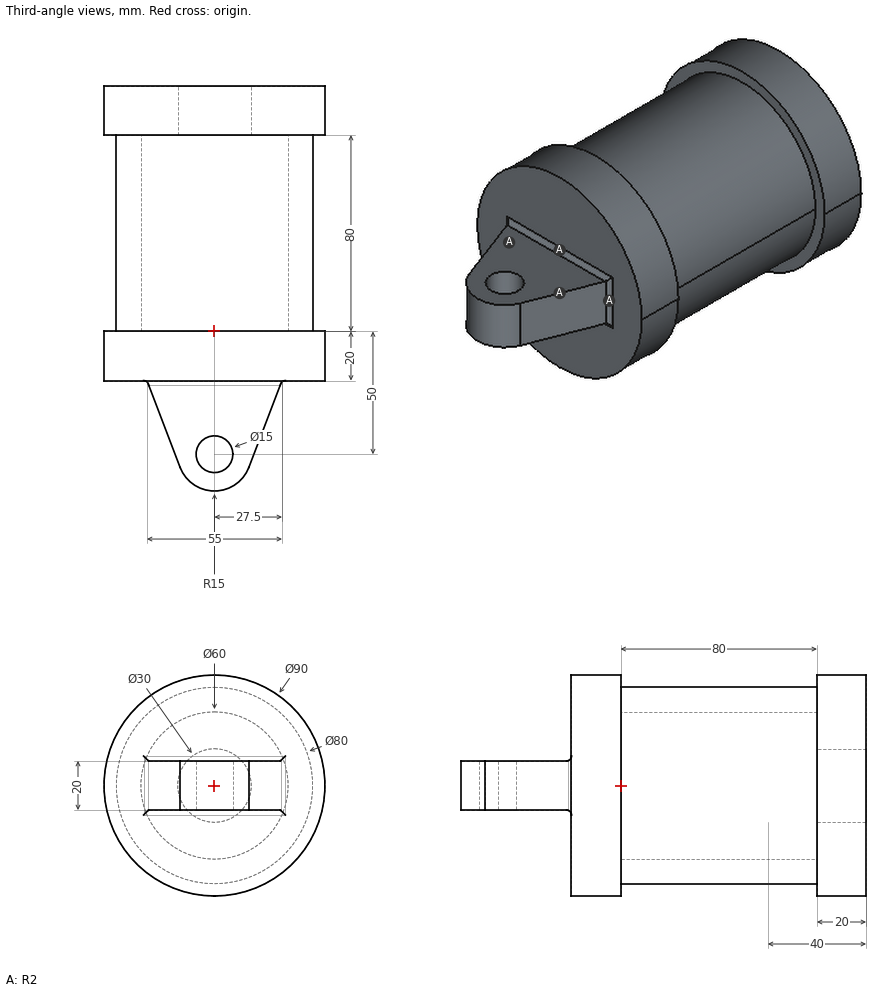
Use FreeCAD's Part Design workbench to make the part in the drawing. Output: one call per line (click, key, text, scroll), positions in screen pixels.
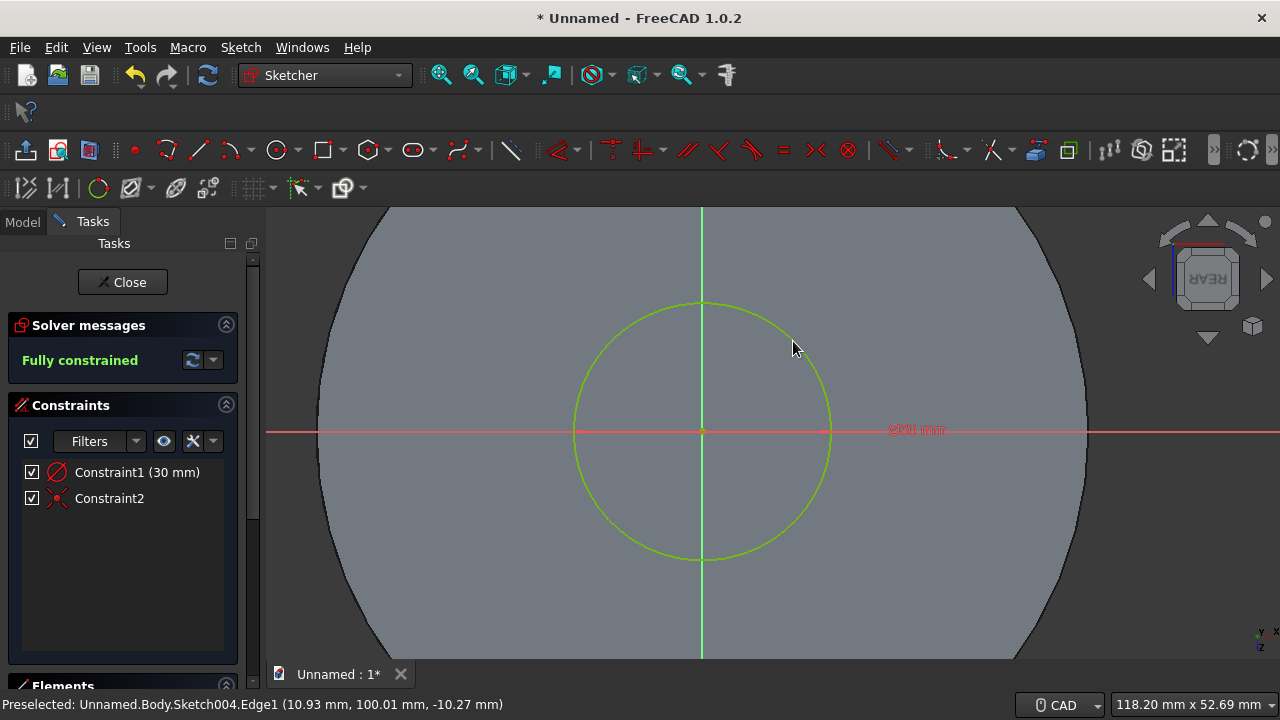
click(123, 282)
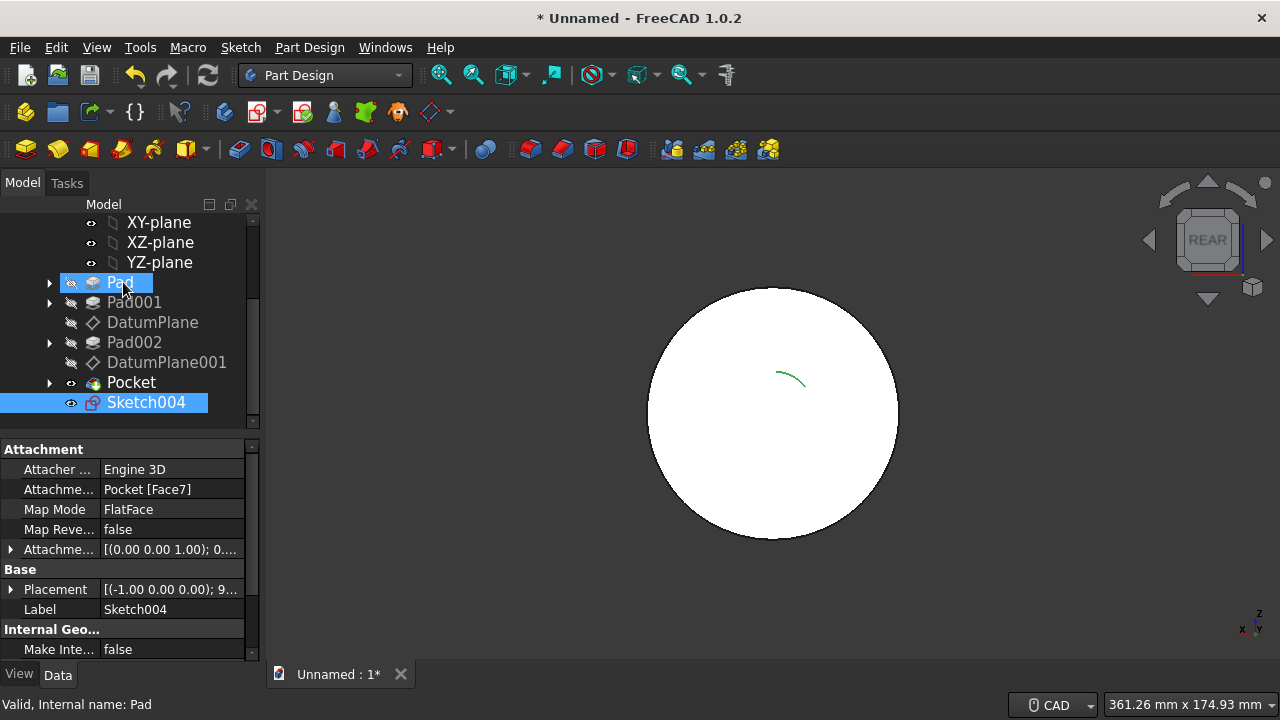
click(240, 150)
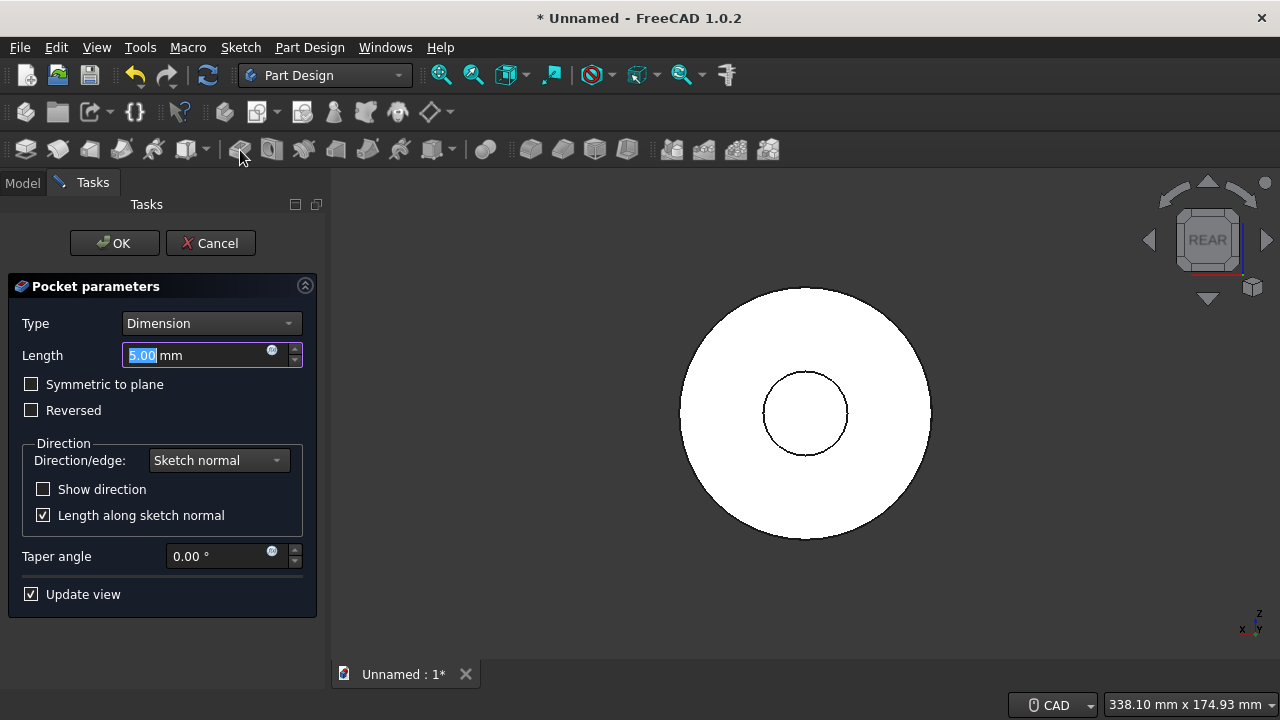
text(40)
key(Tab)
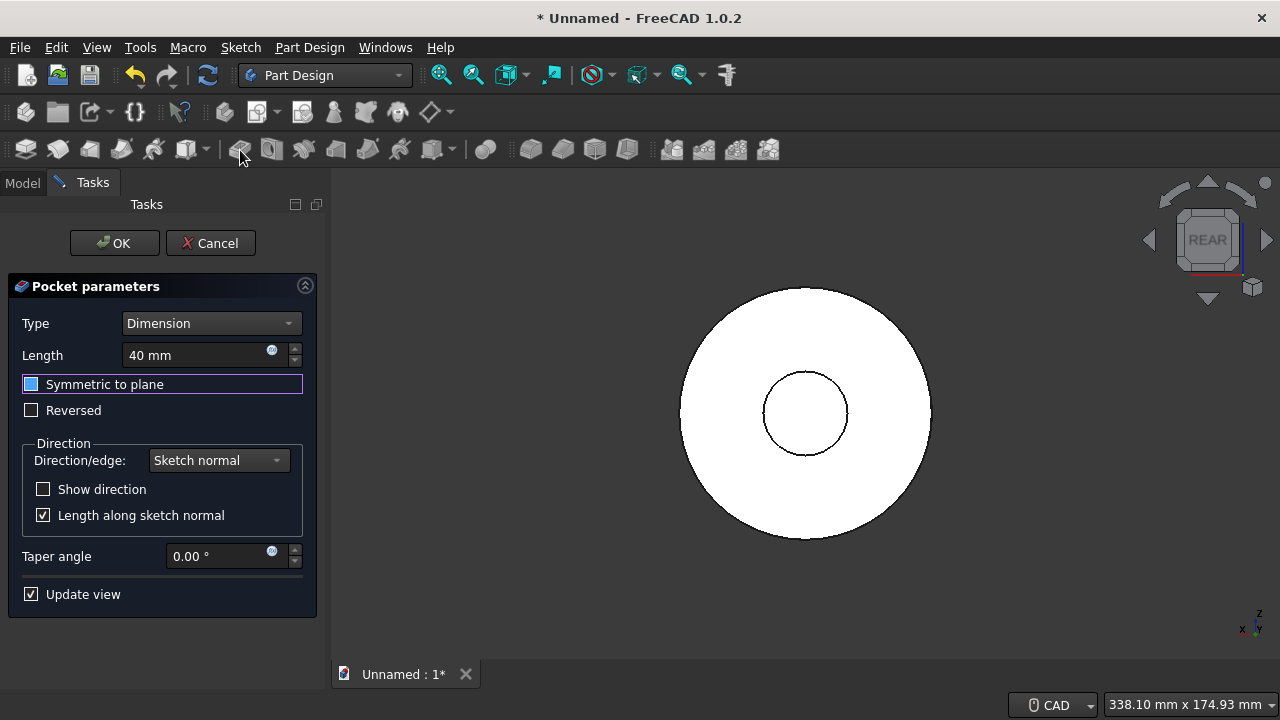
click(115, 243)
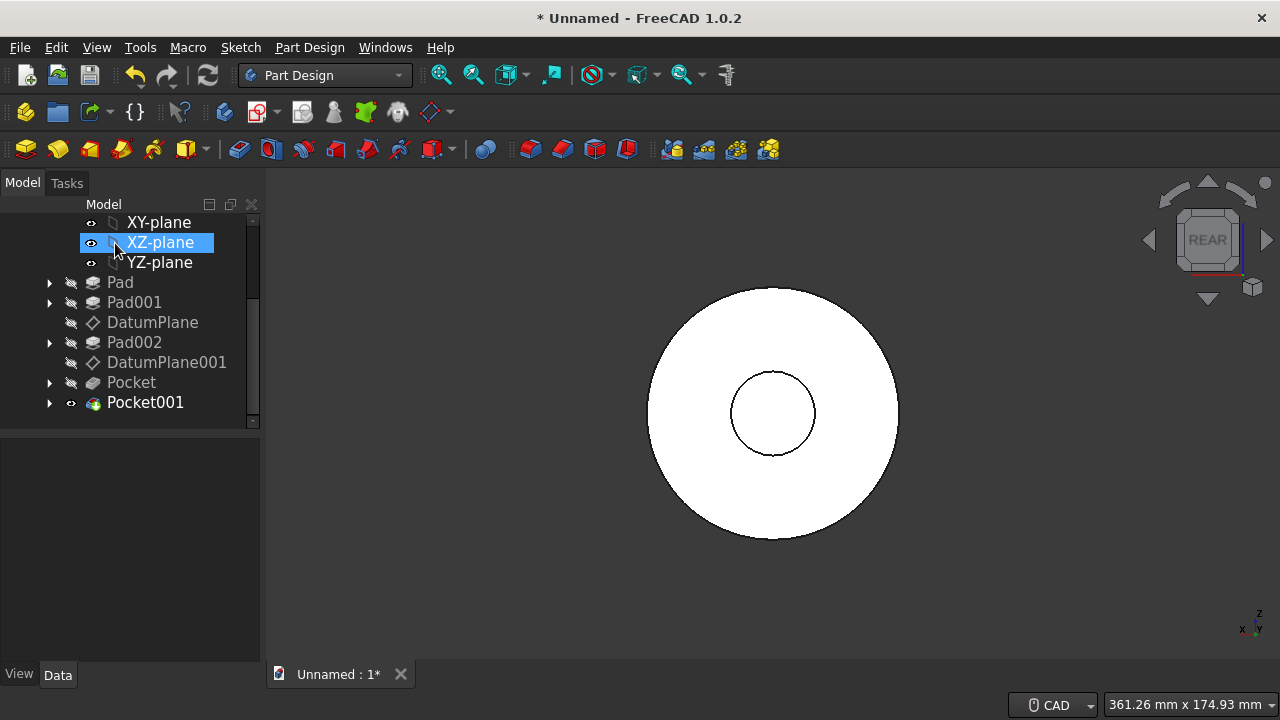
click(258, 112)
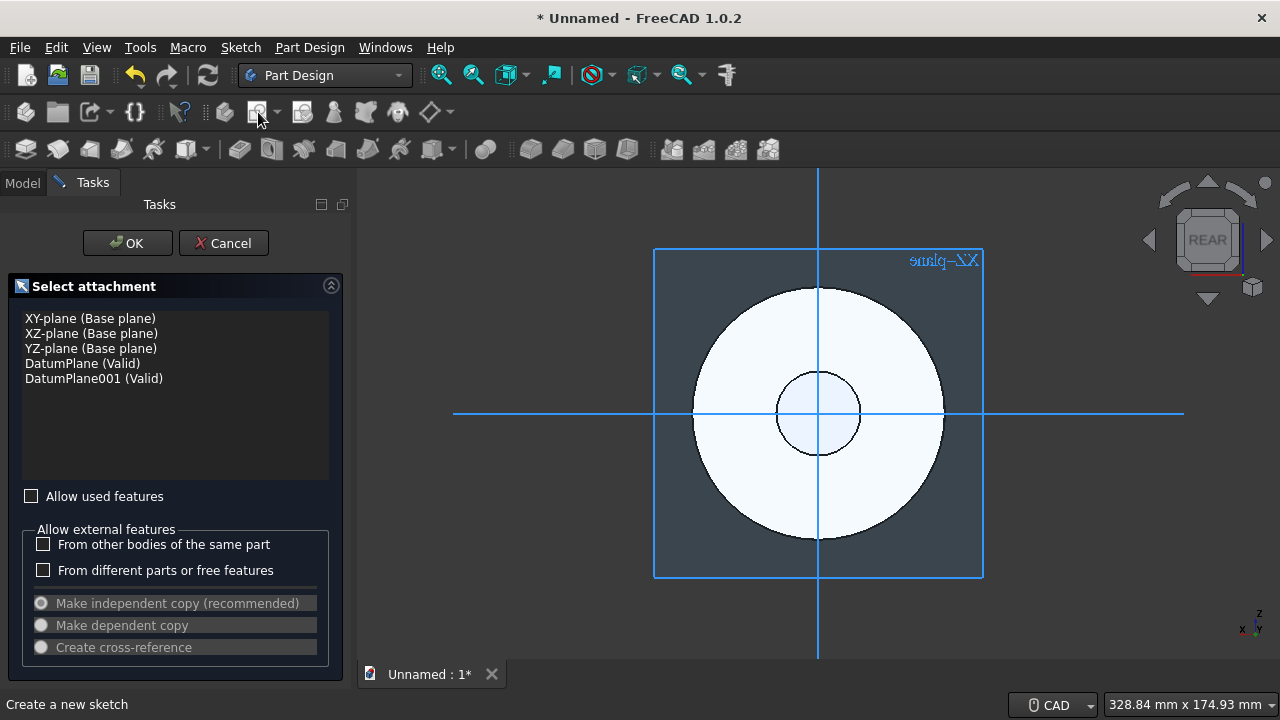
click(82, 318)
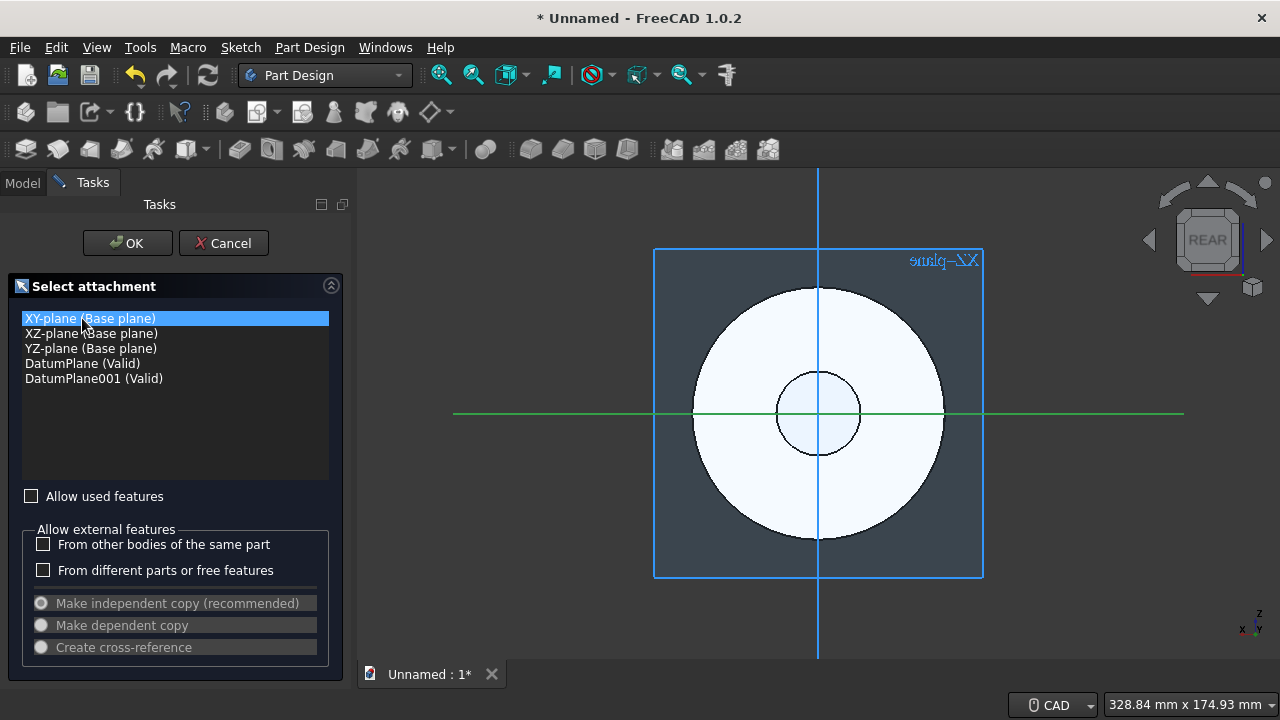
click(128, 243)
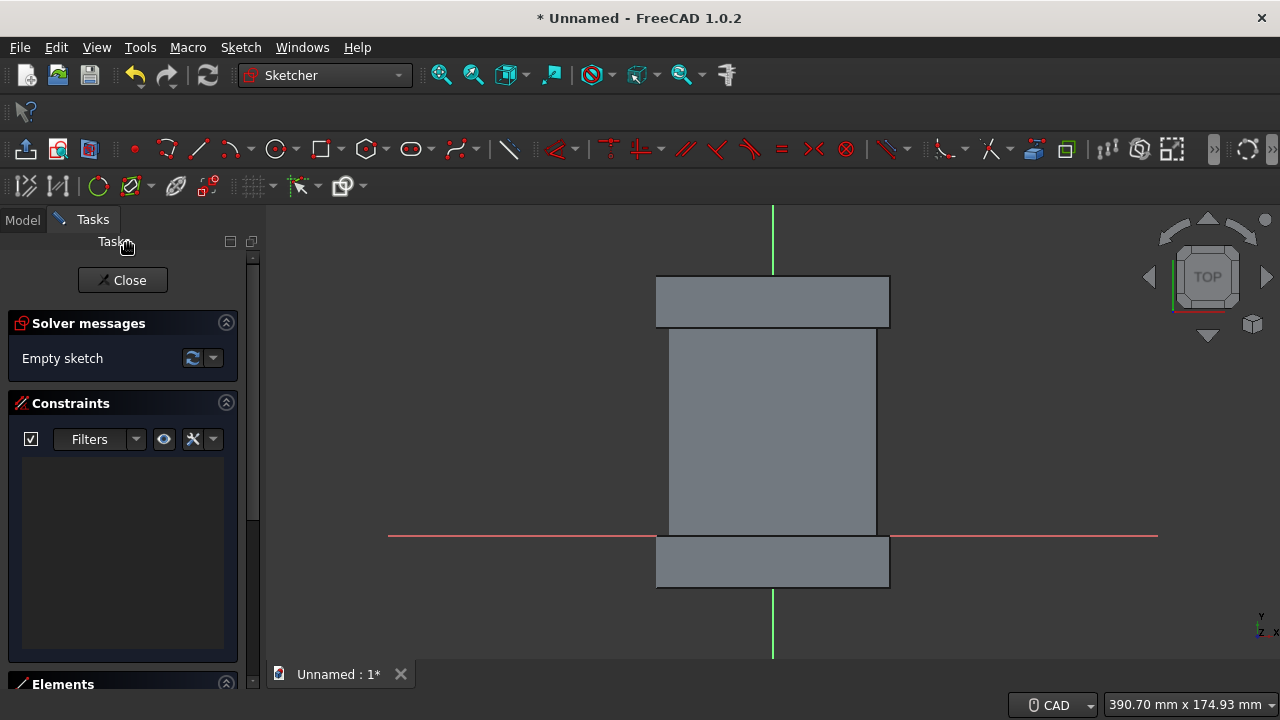
click(90, 150)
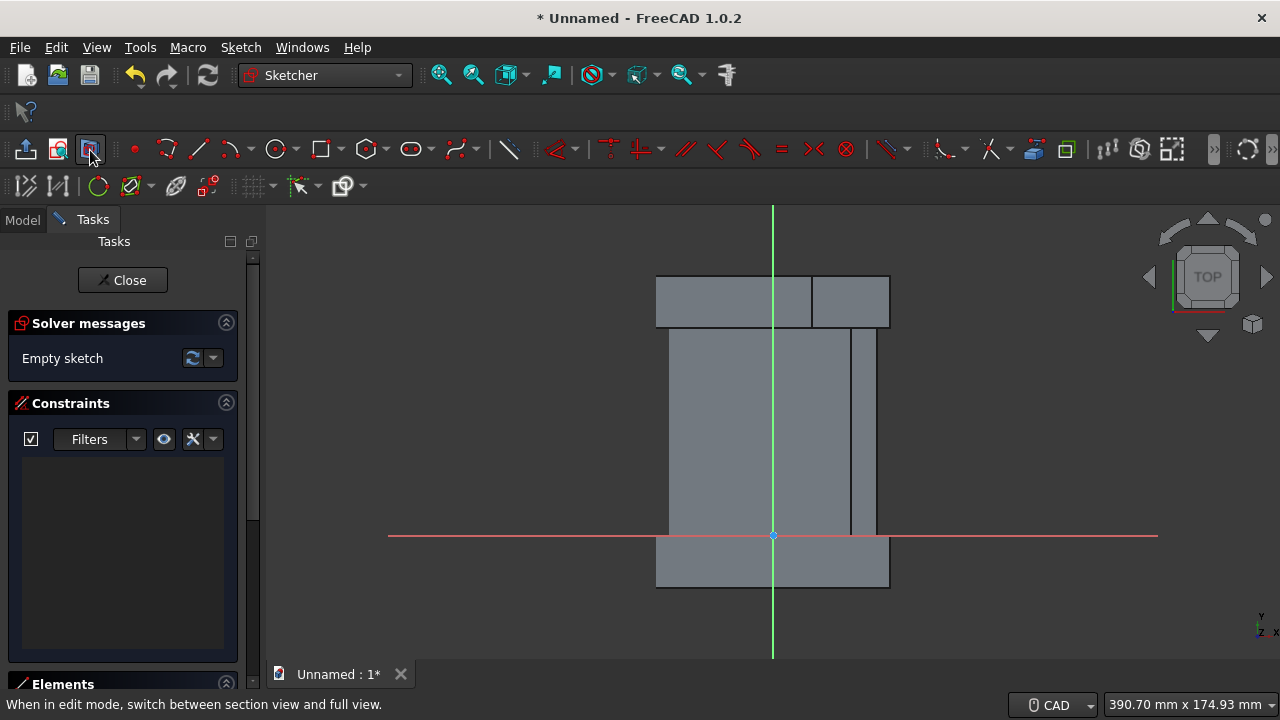
scroll(704, 432, down, 5)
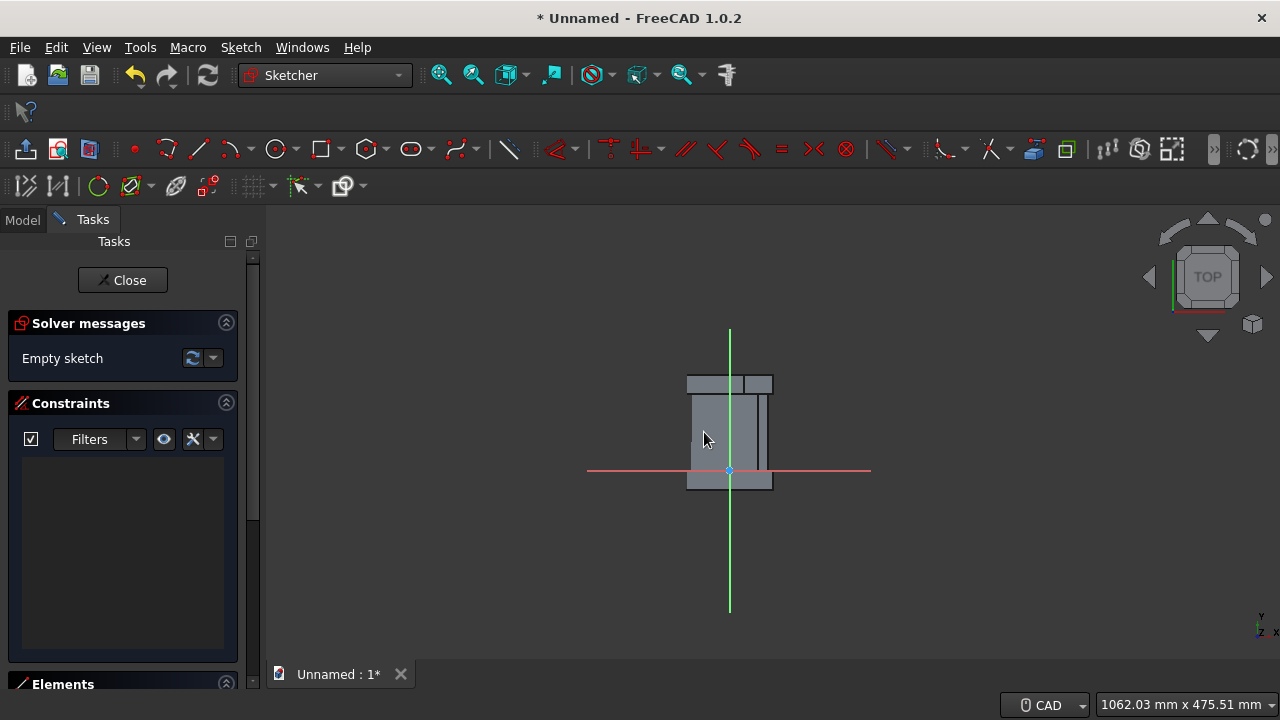
scroll(736, 519, up, 8)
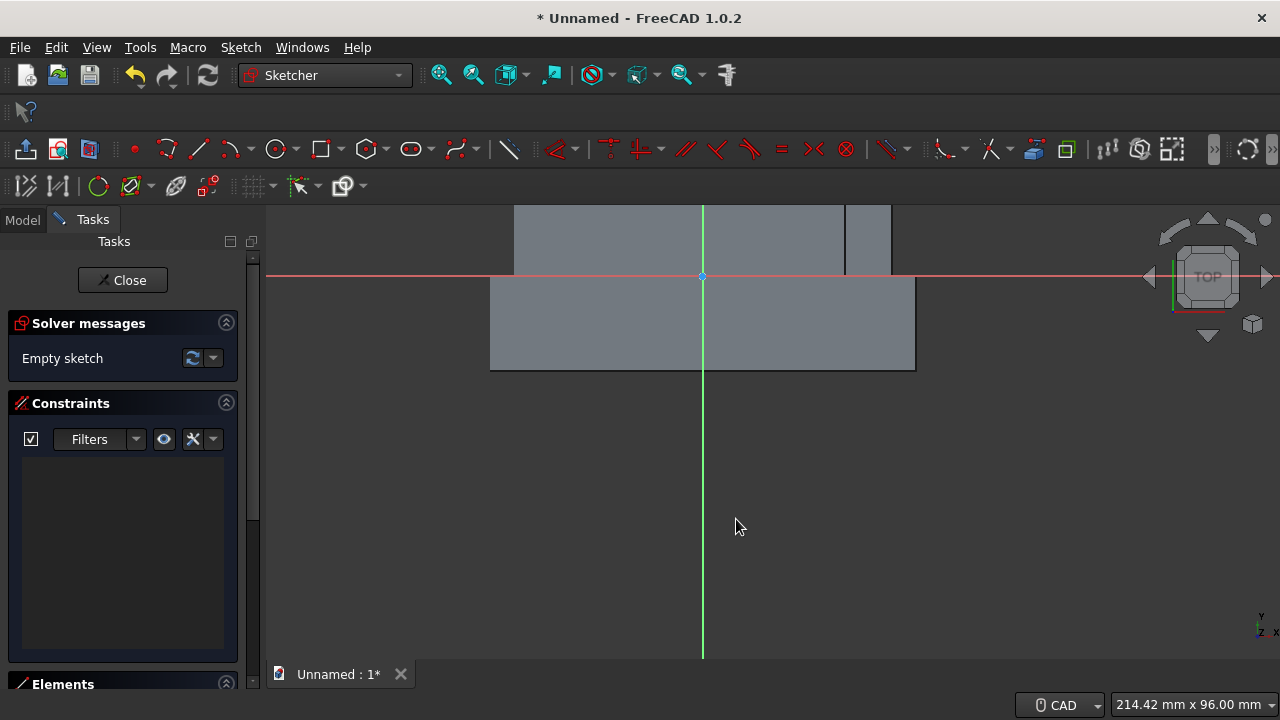
click(168, 150)